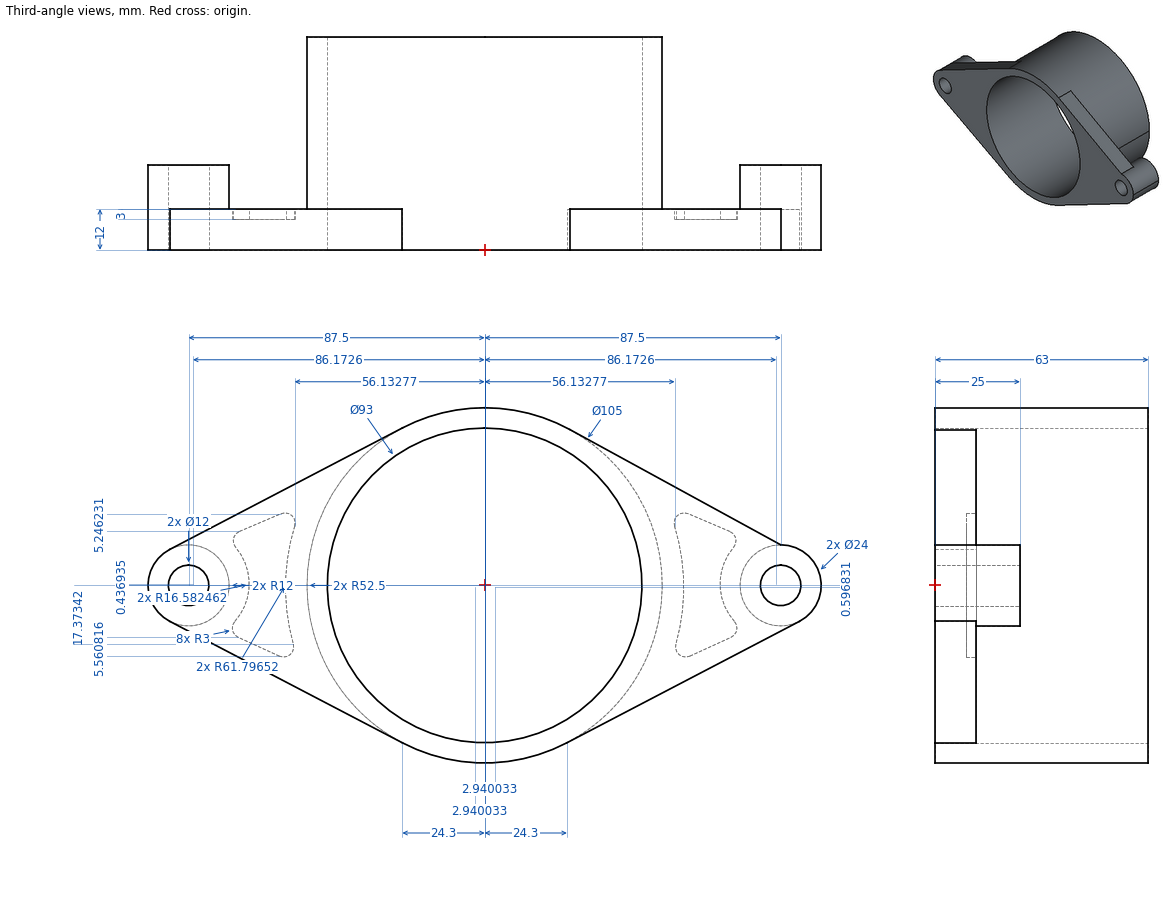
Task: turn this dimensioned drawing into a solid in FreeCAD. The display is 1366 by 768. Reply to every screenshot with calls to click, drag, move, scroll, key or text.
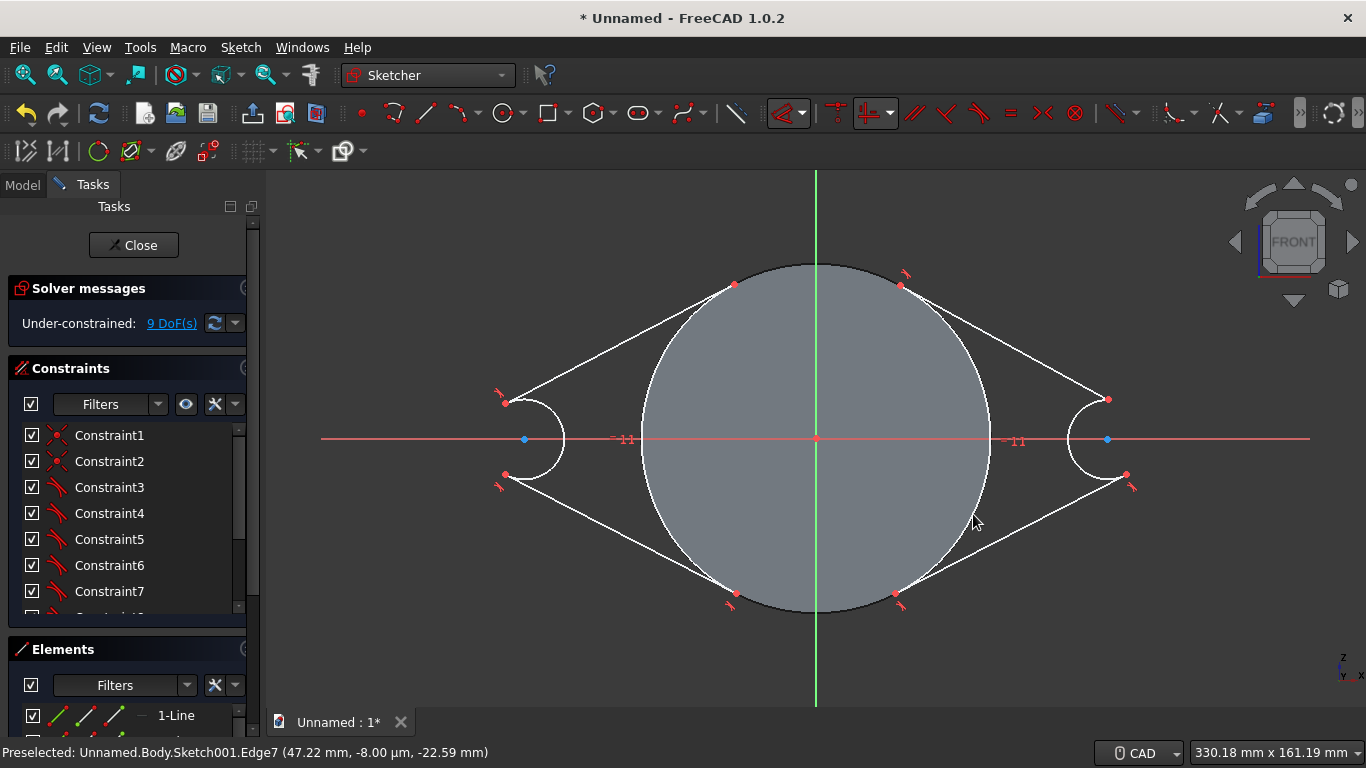
click(552, 469)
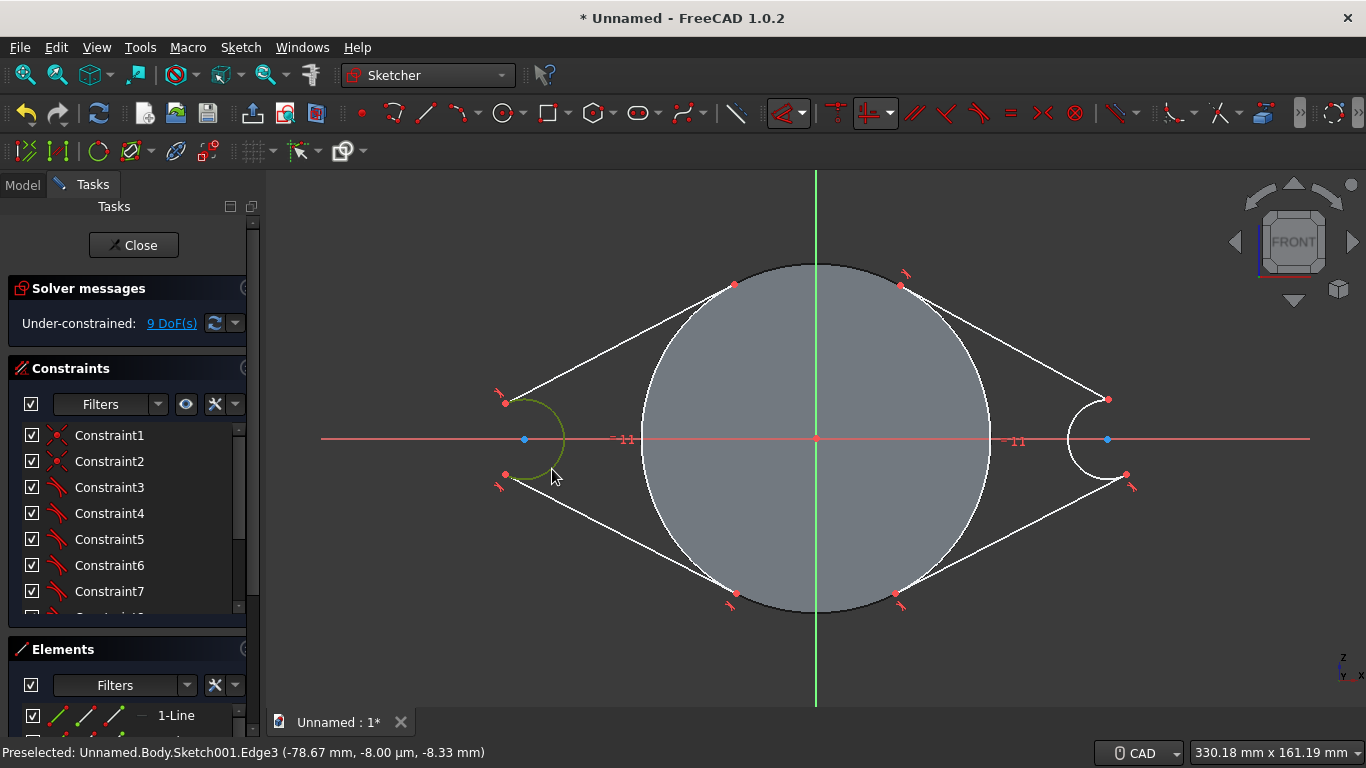
click(1073, 421)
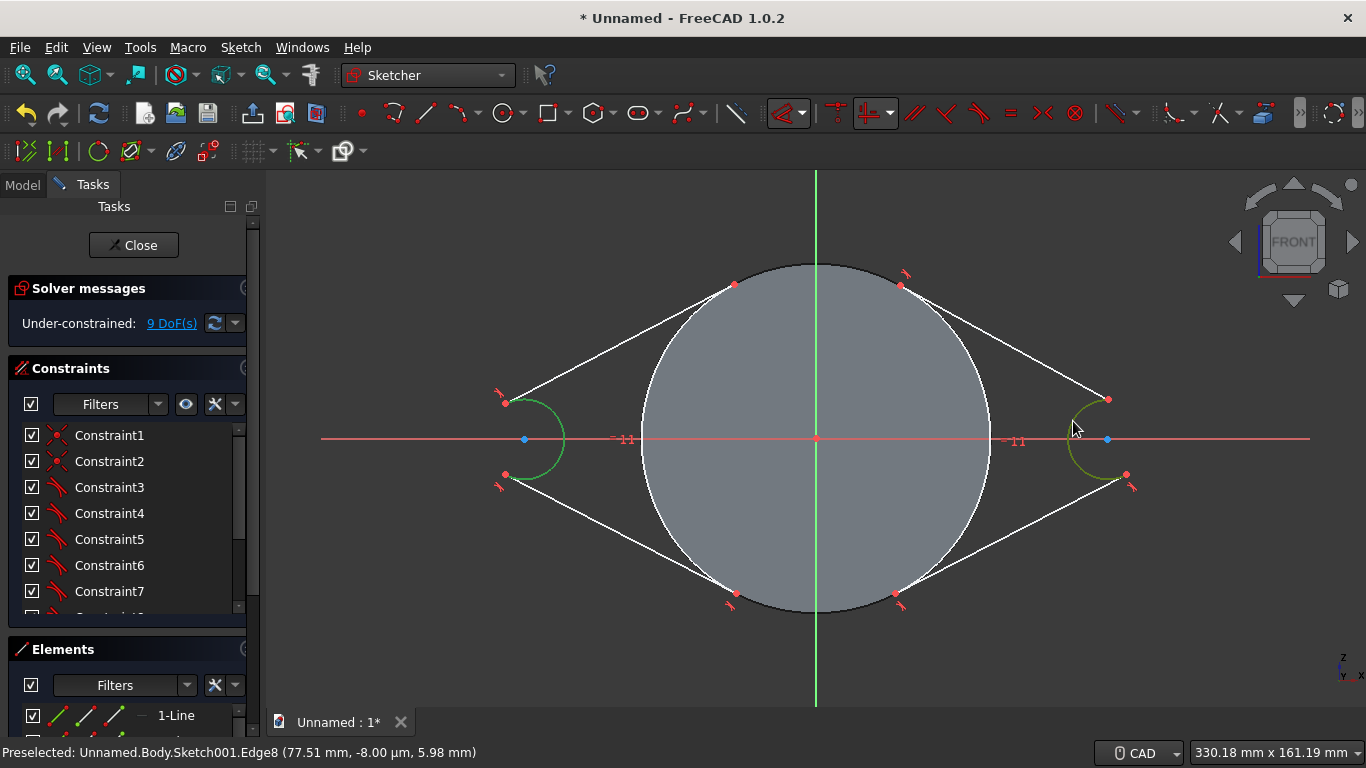
click(1012, 114)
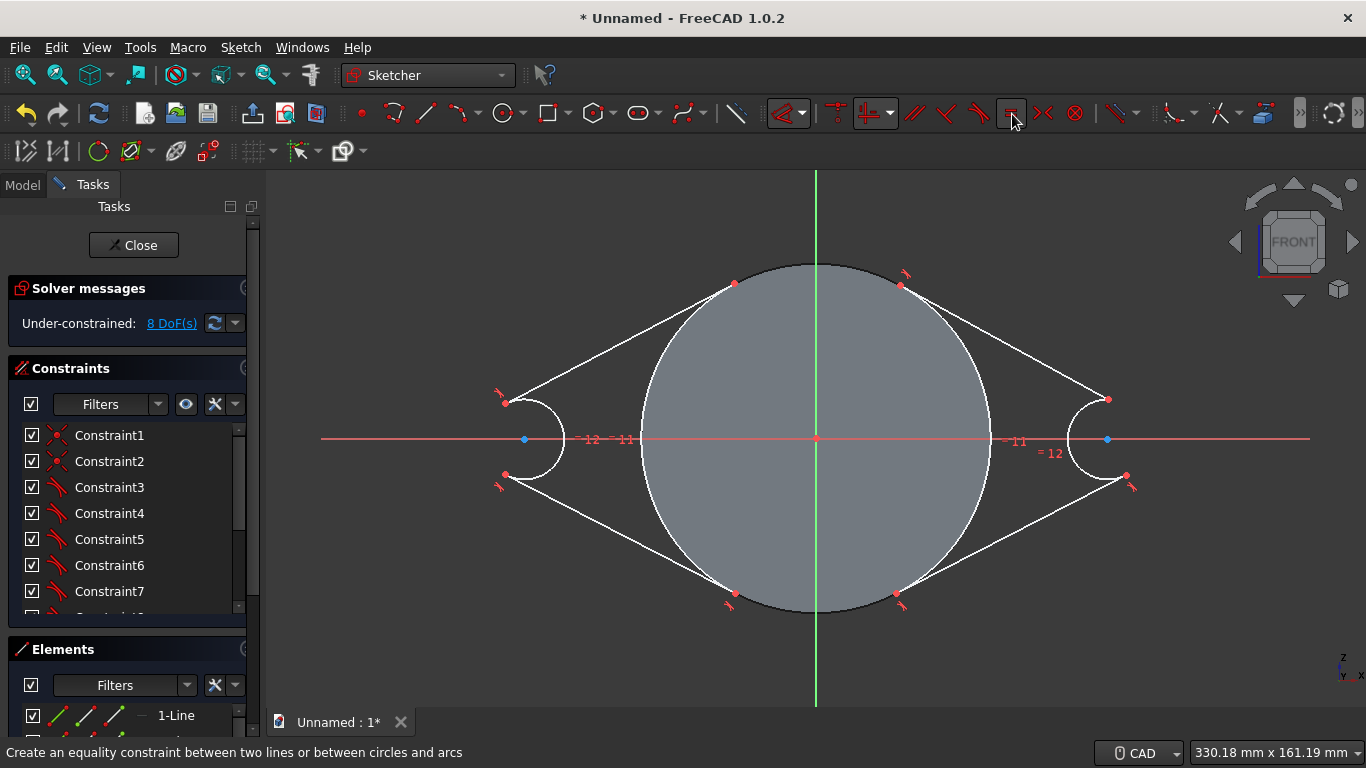
click(524, 439)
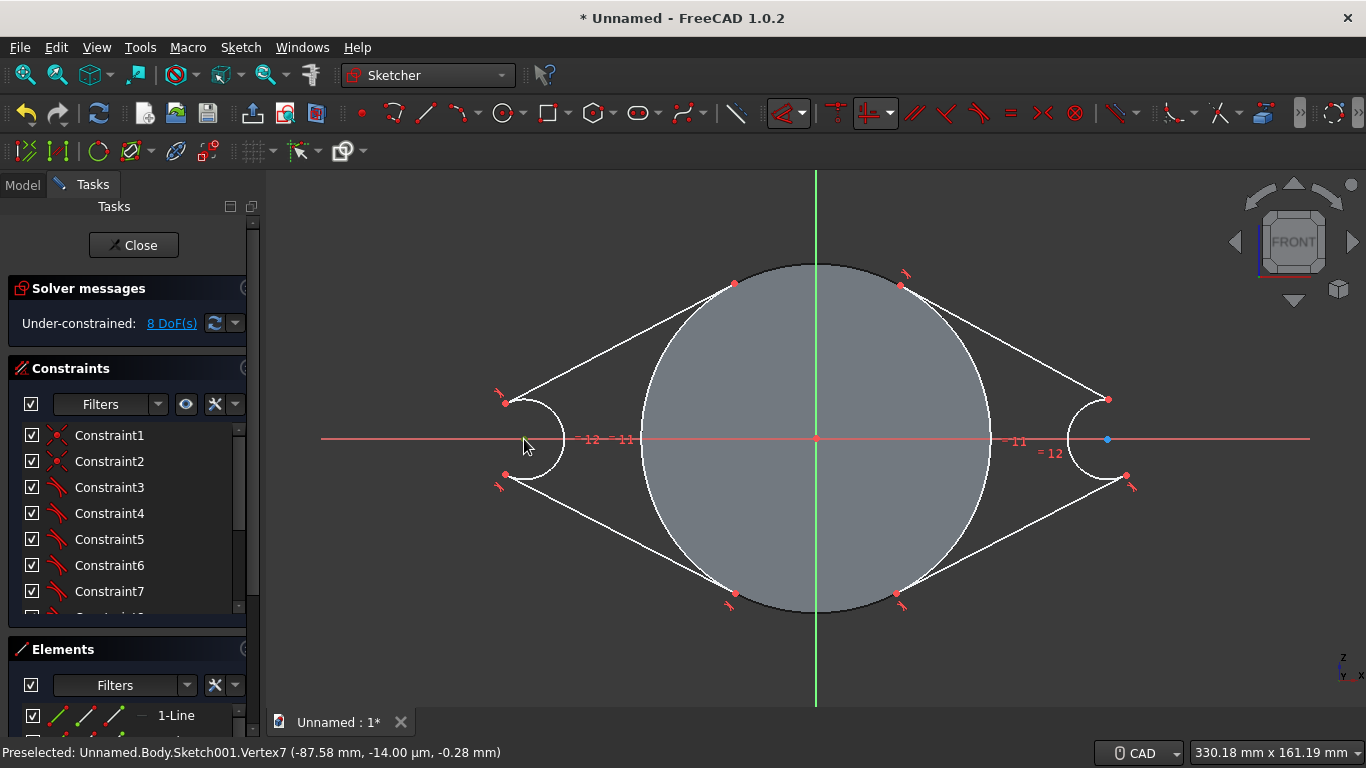
click(359, 439)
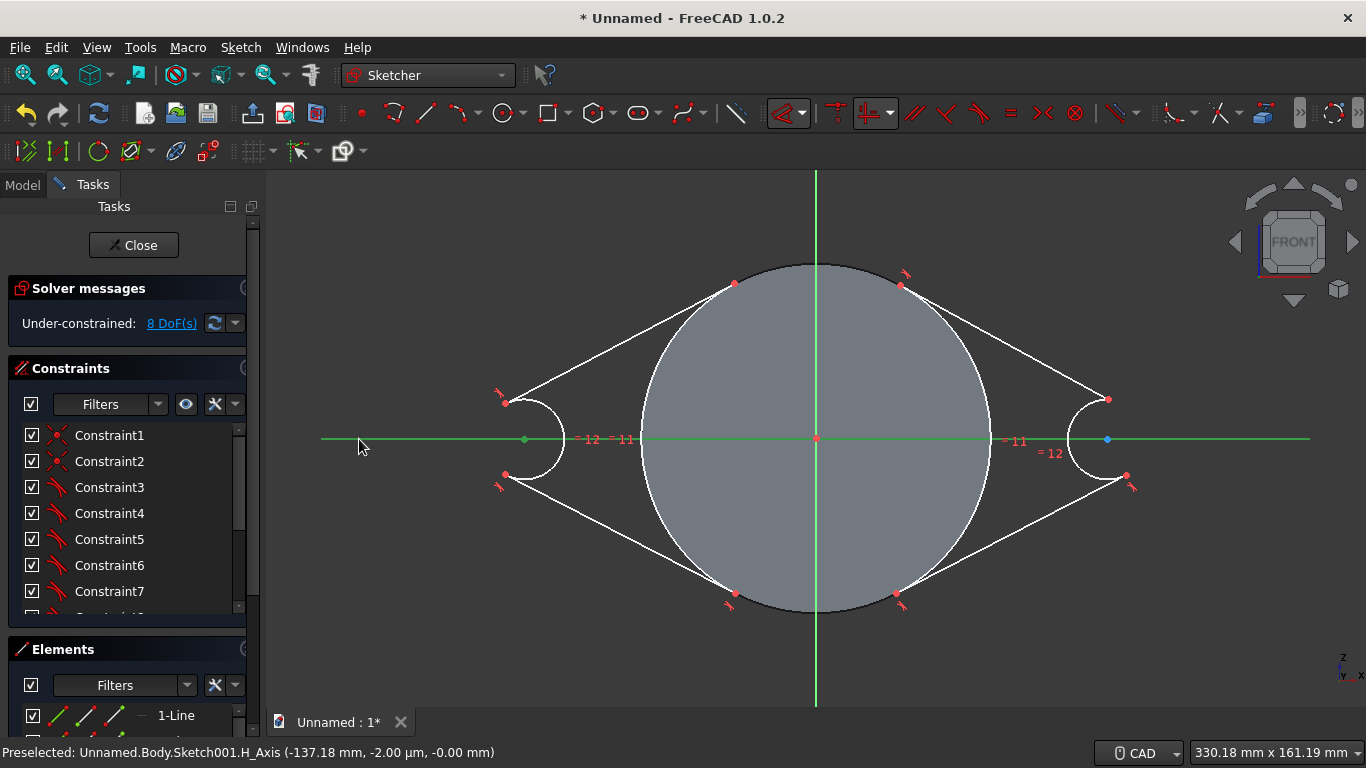
click(836, 114)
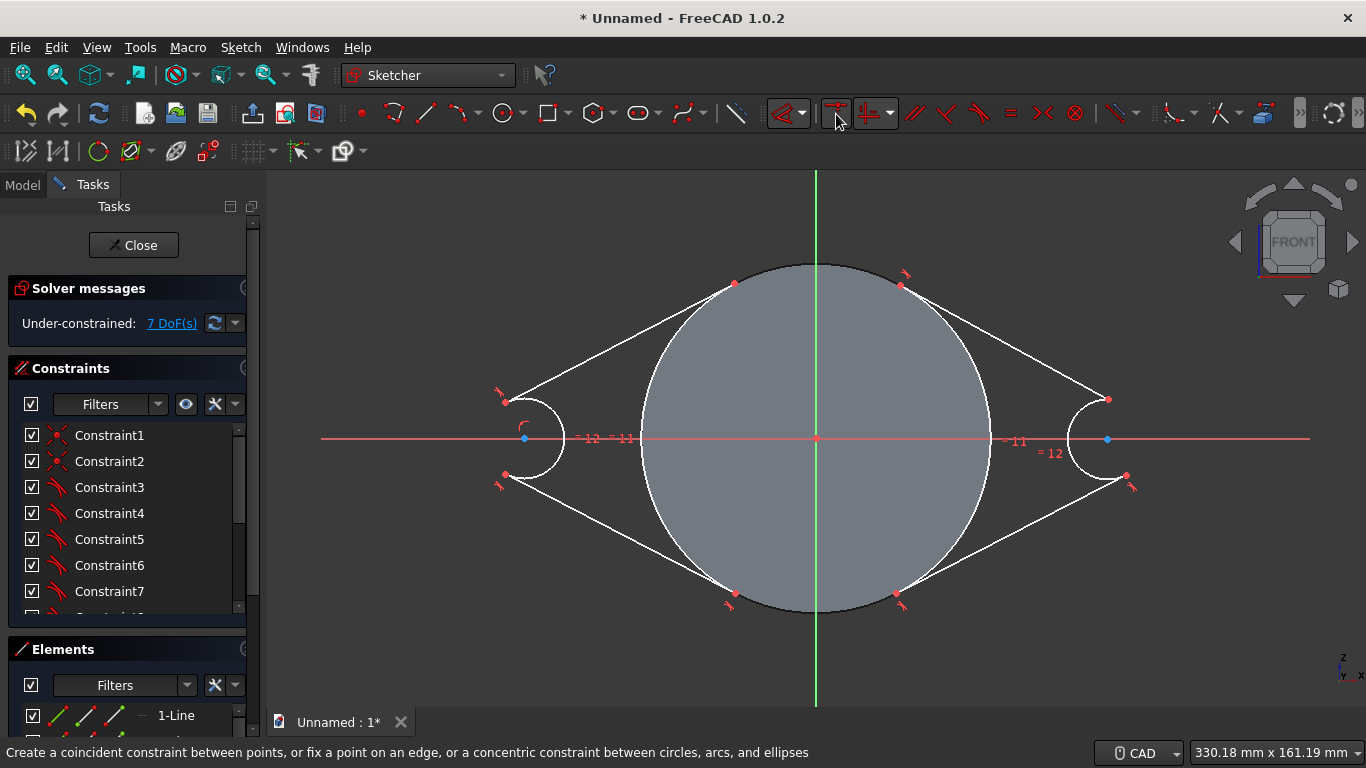
click(1108, 439)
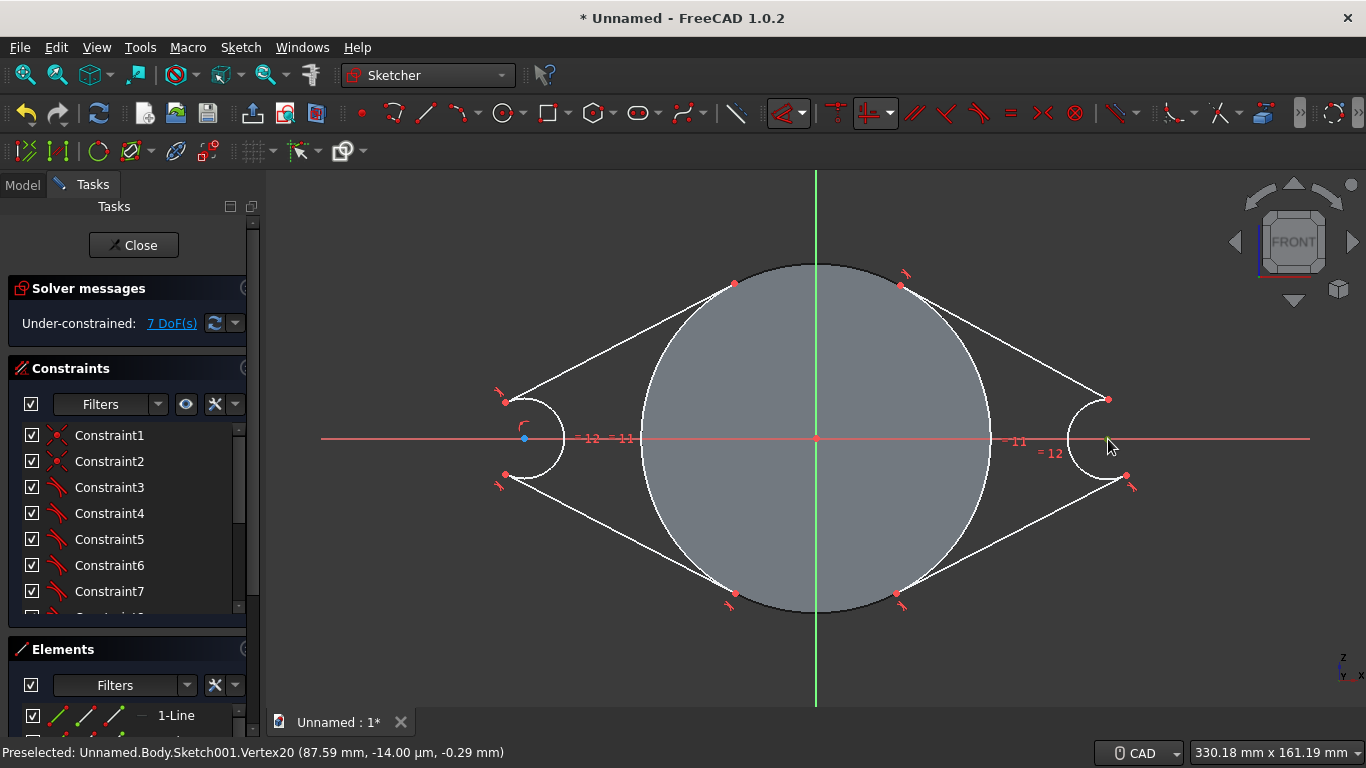
click(359, 439)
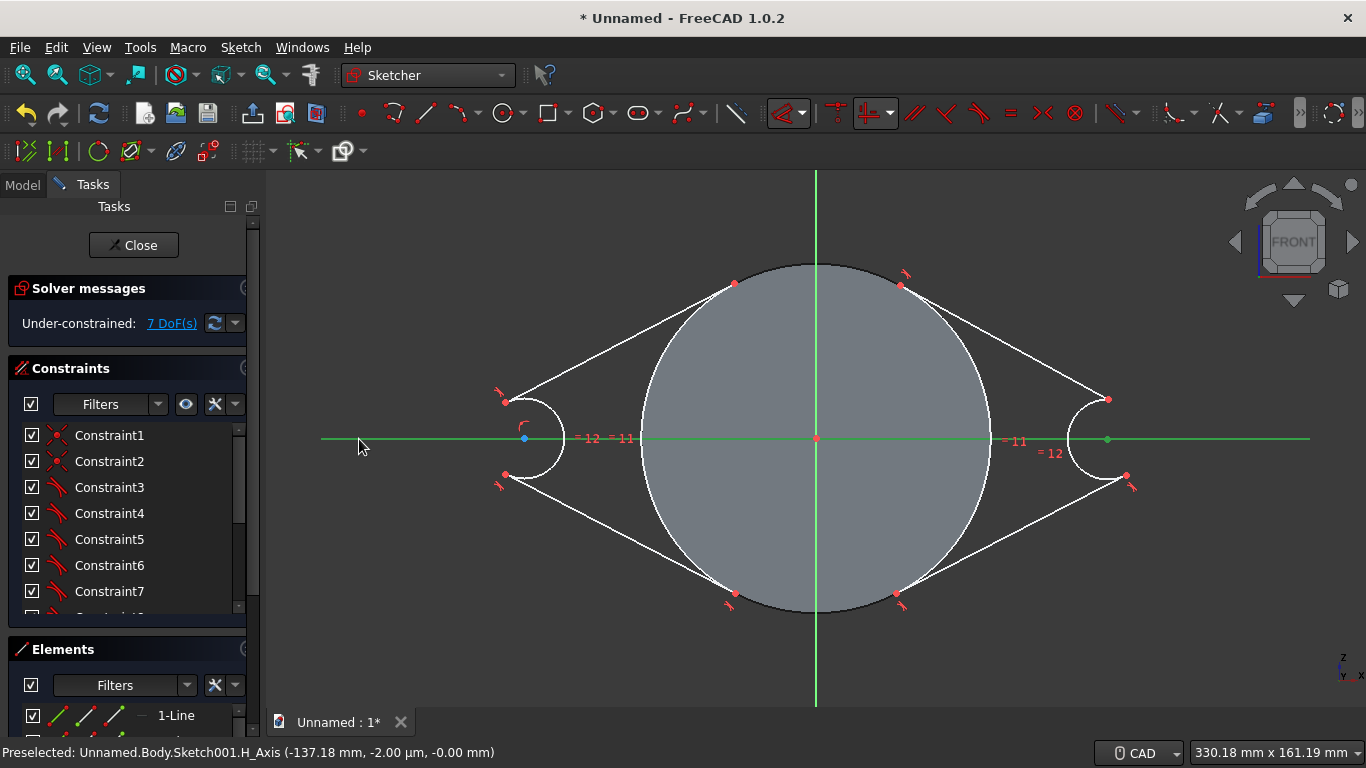
key(c)